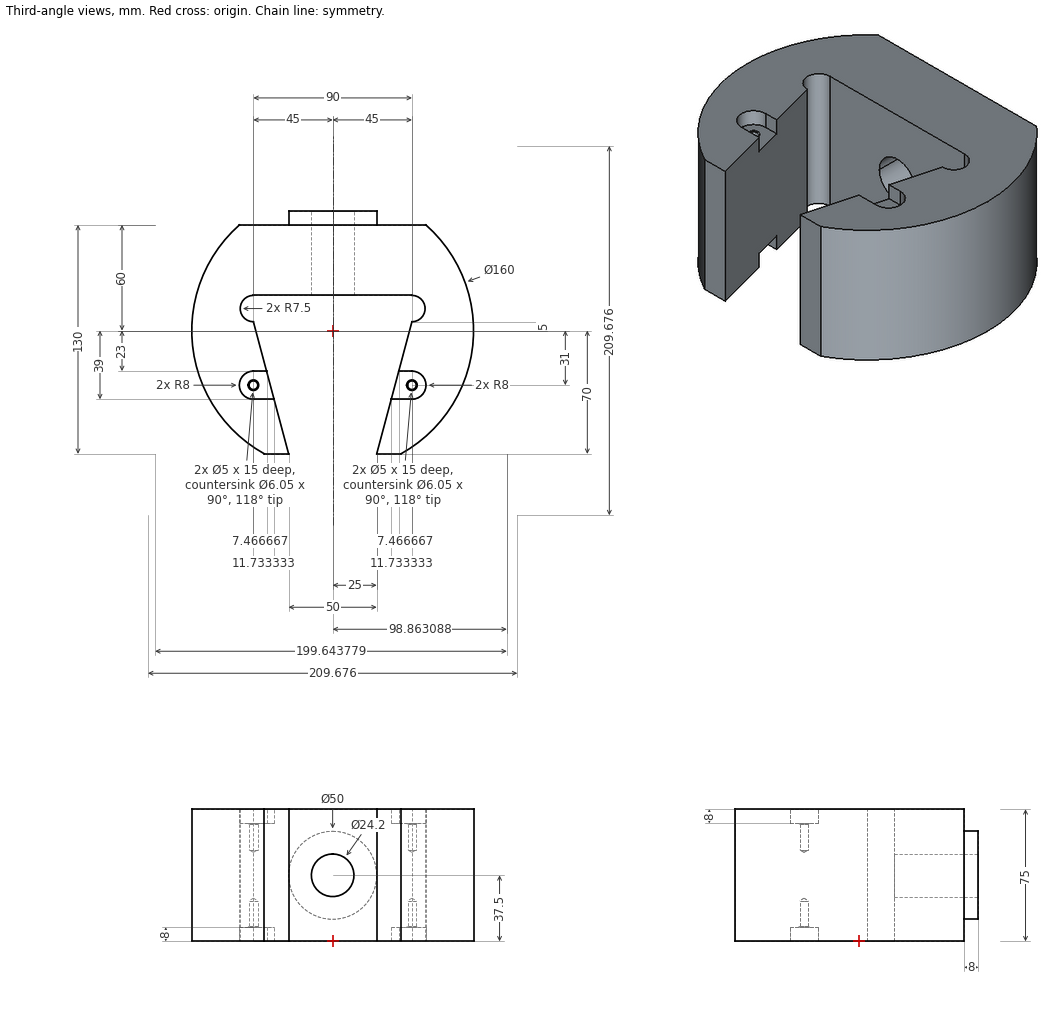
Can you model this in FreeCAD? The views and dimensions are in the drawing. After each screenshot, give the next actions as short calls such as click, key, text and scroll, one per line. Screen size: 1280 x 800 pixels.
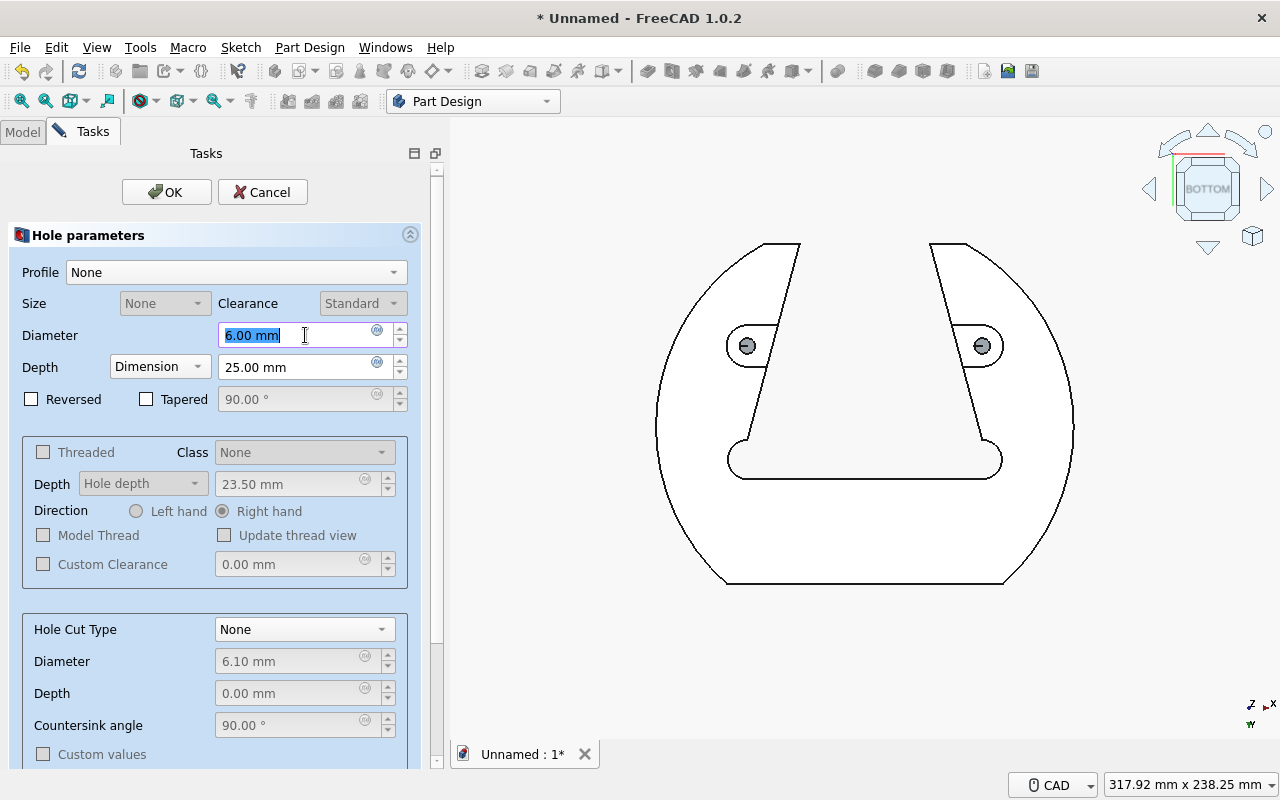
text(5)
key(Tab)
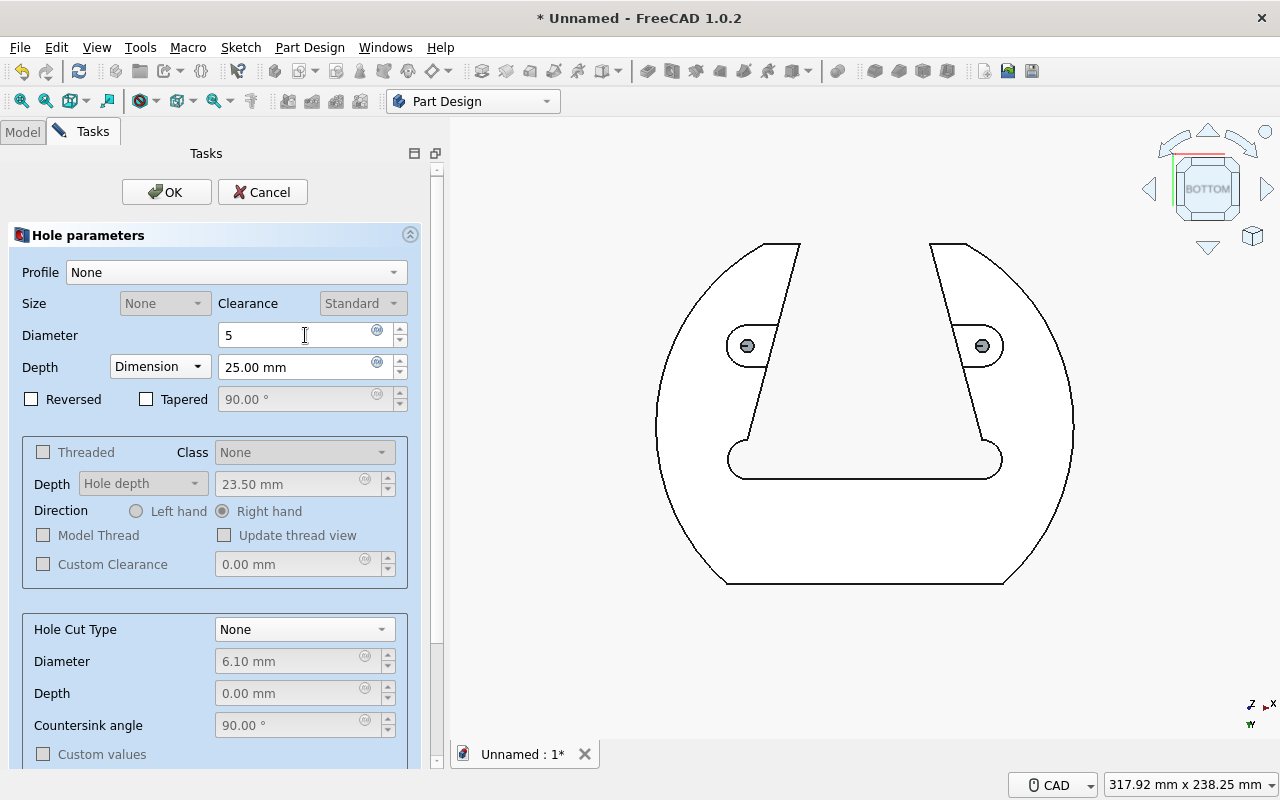
triple_click(305, 367)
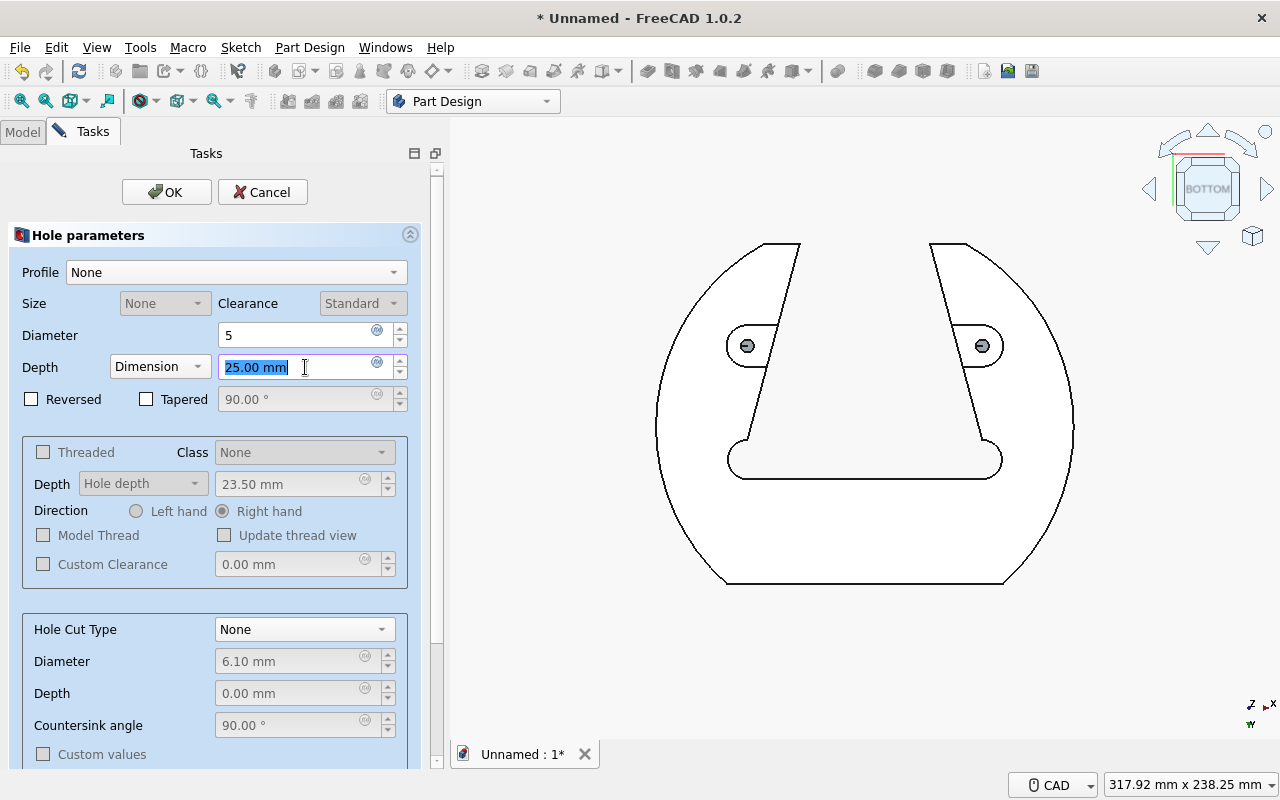
text(15)
key(Tab)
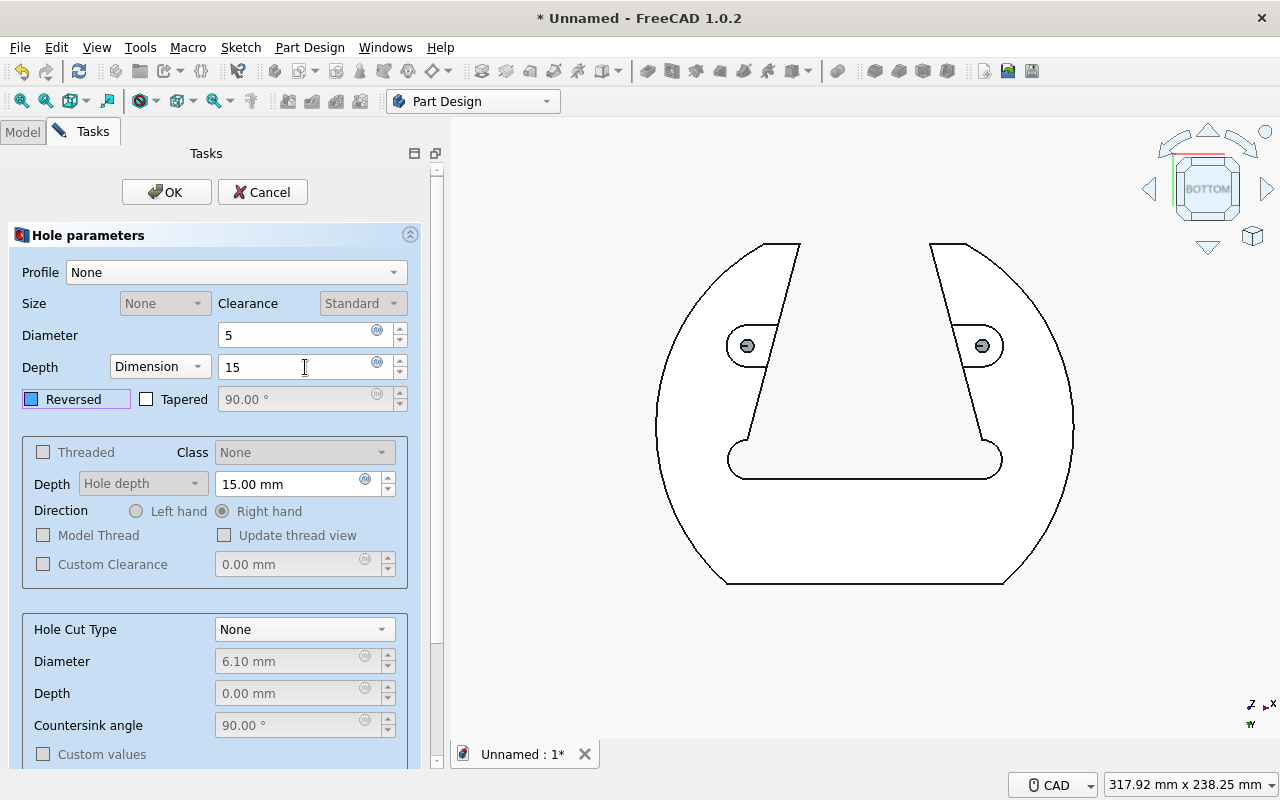
click(306, 630)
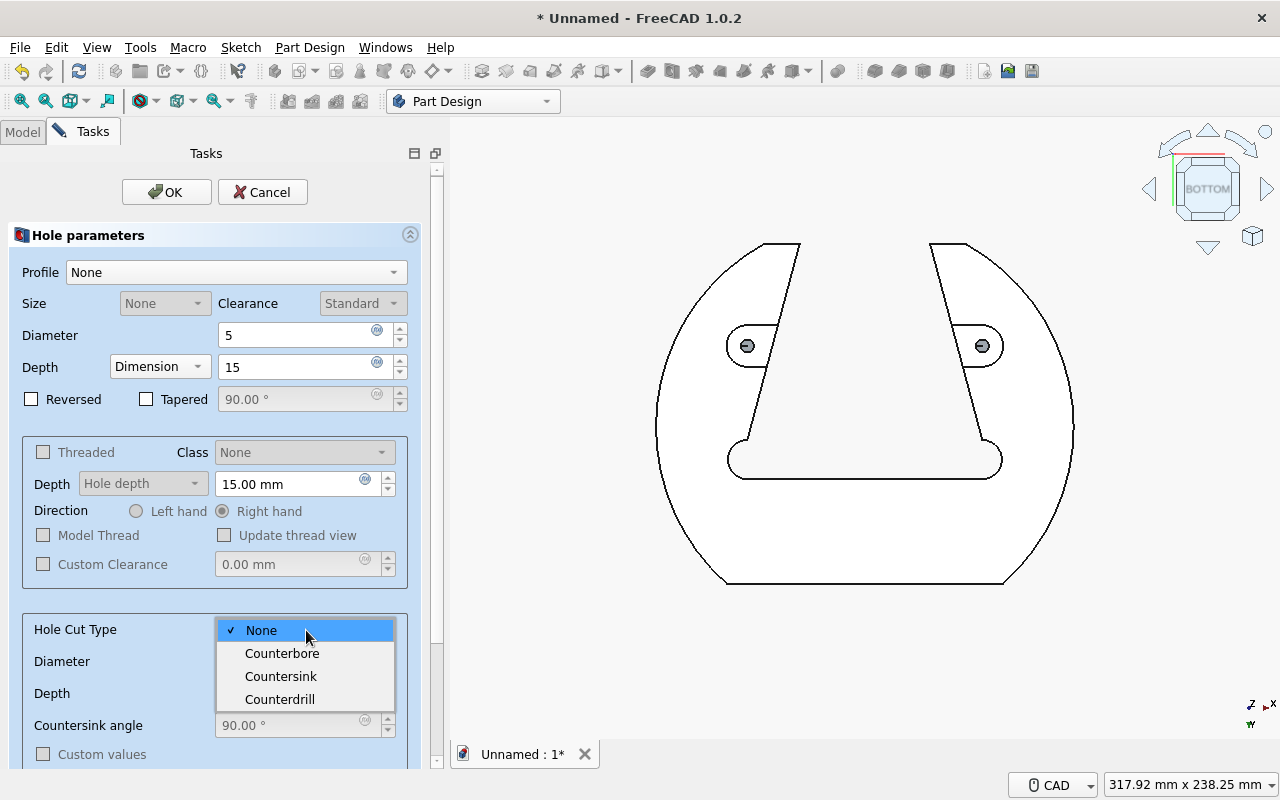
click(304, 676)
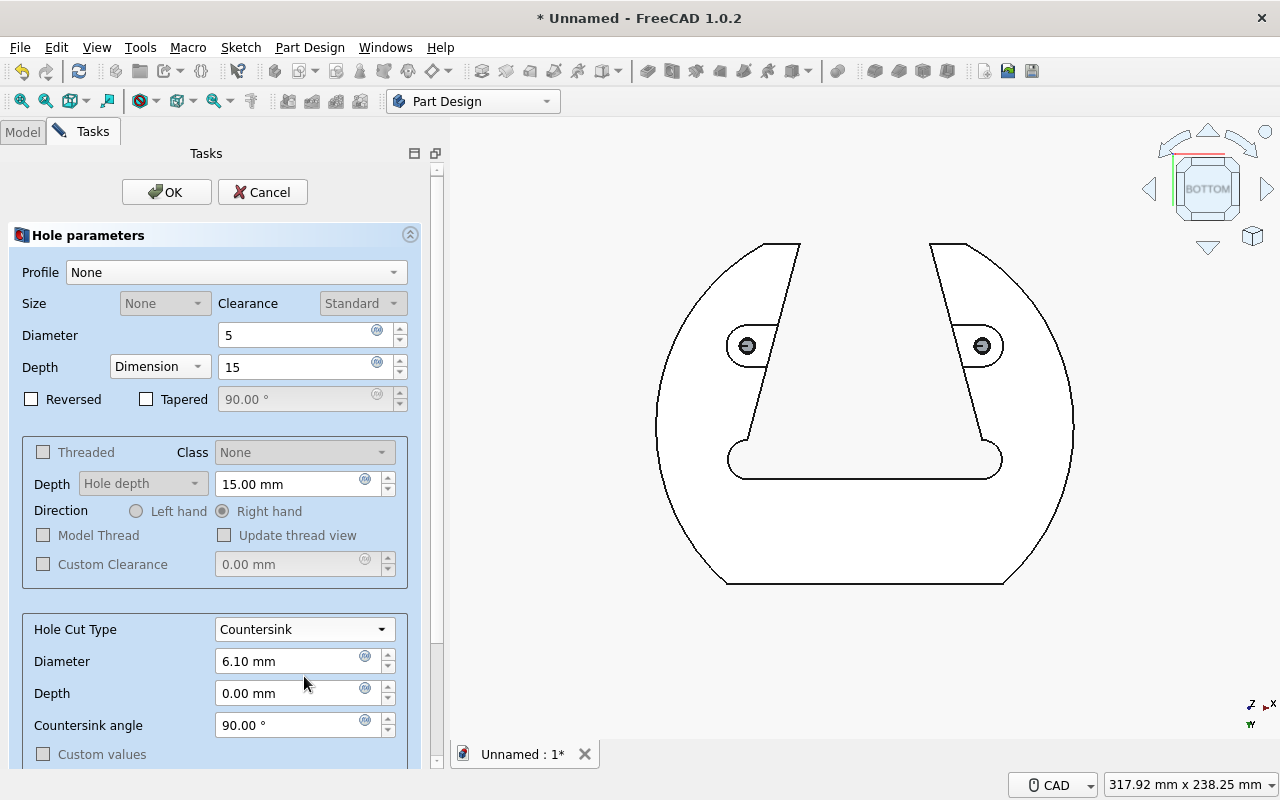
triple_click(298, 661)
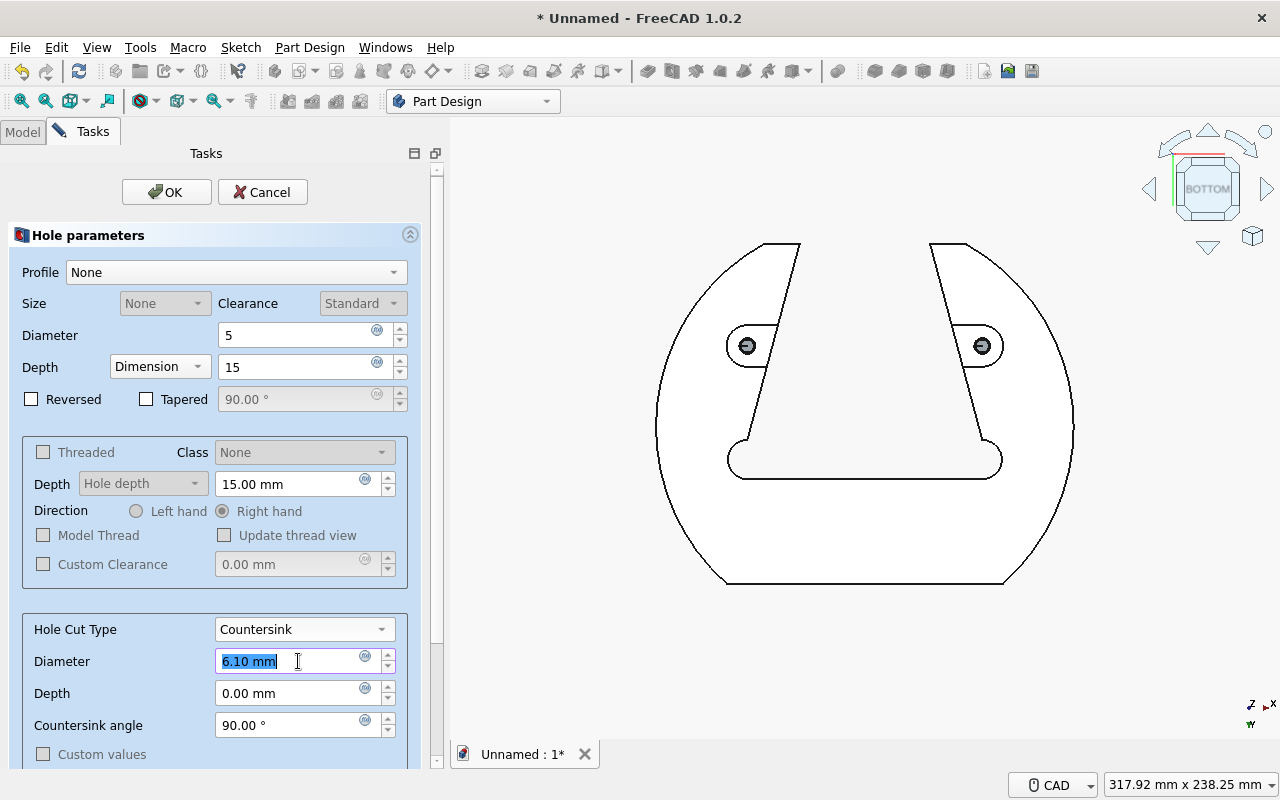
text(6.05)
key(Tab)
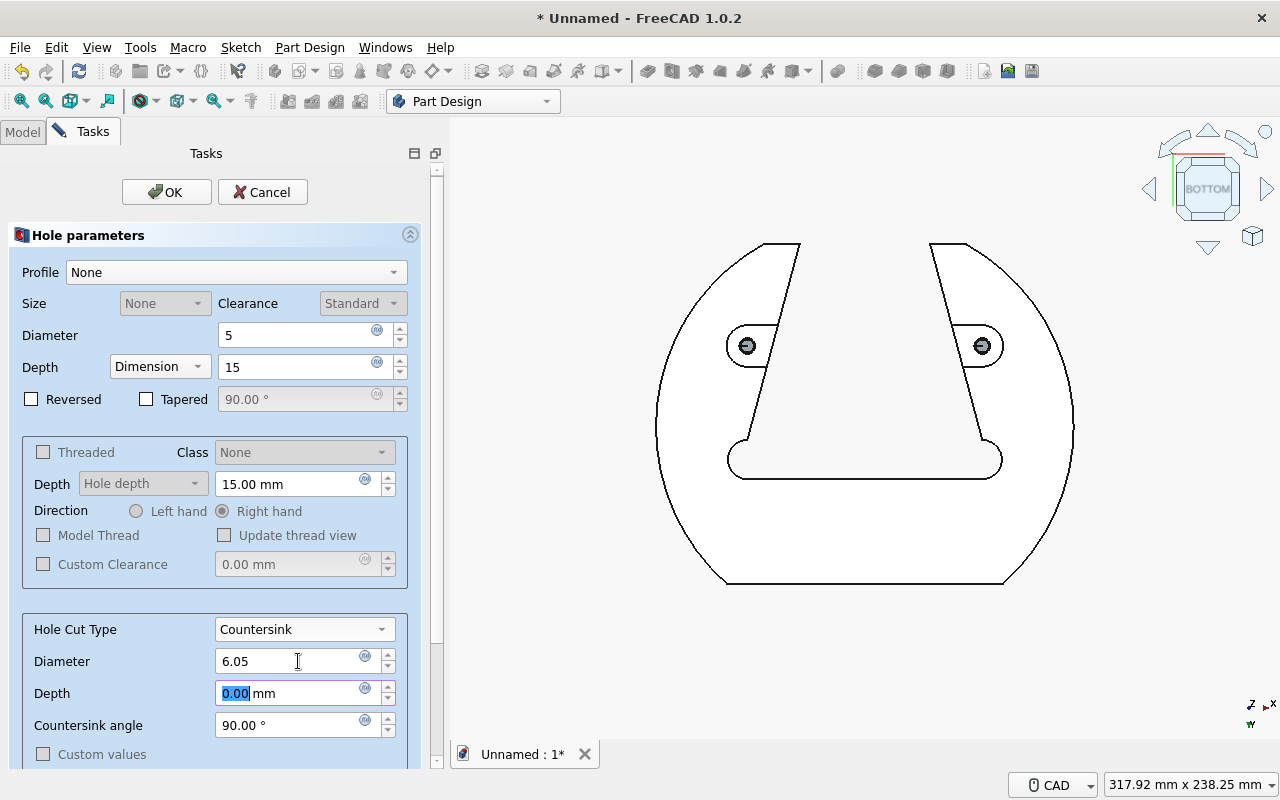
click(167, 192)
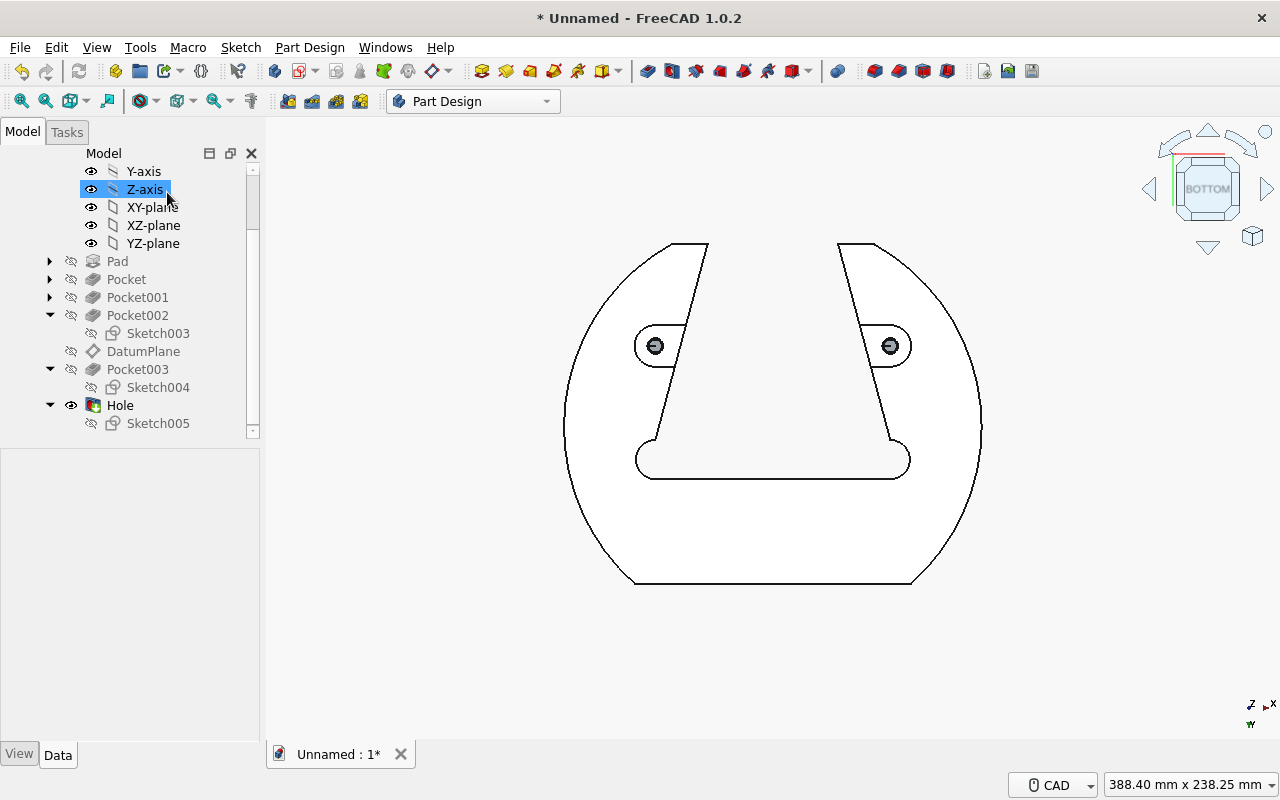
key(0)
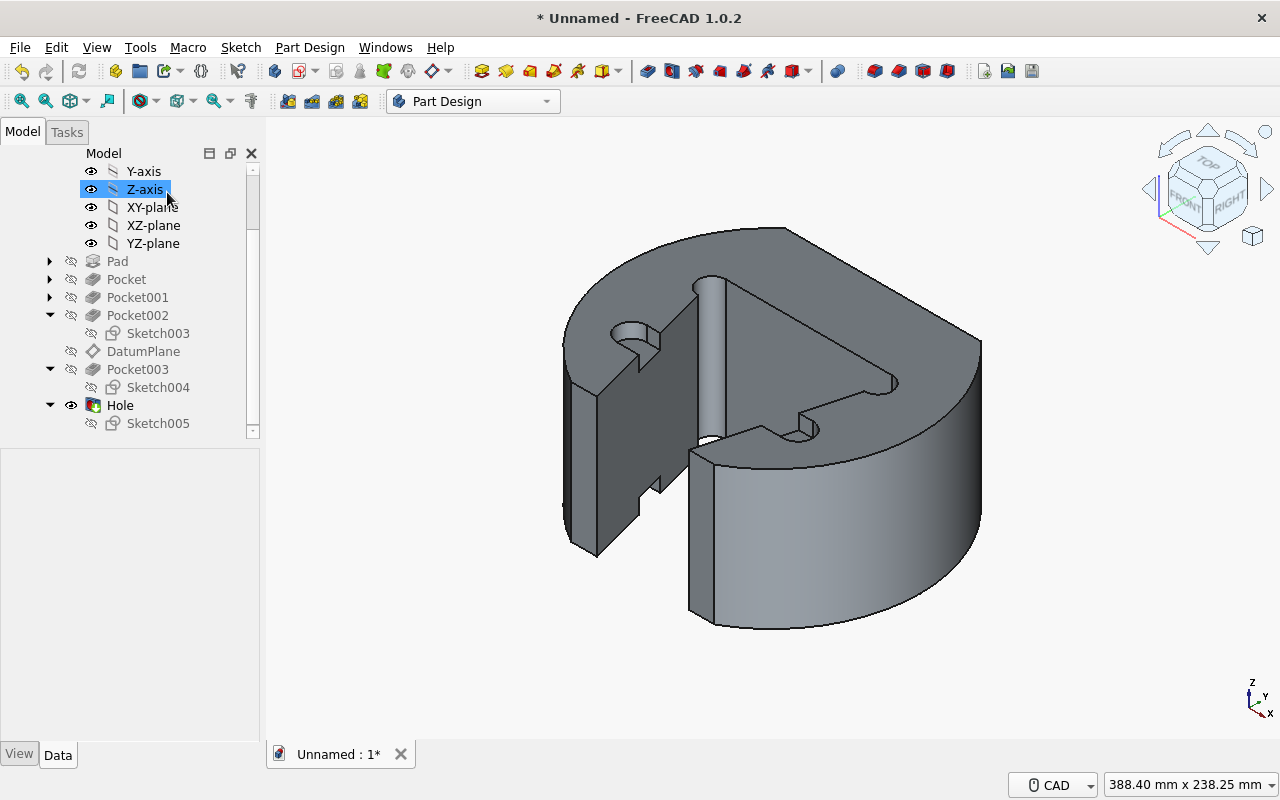
key(2)